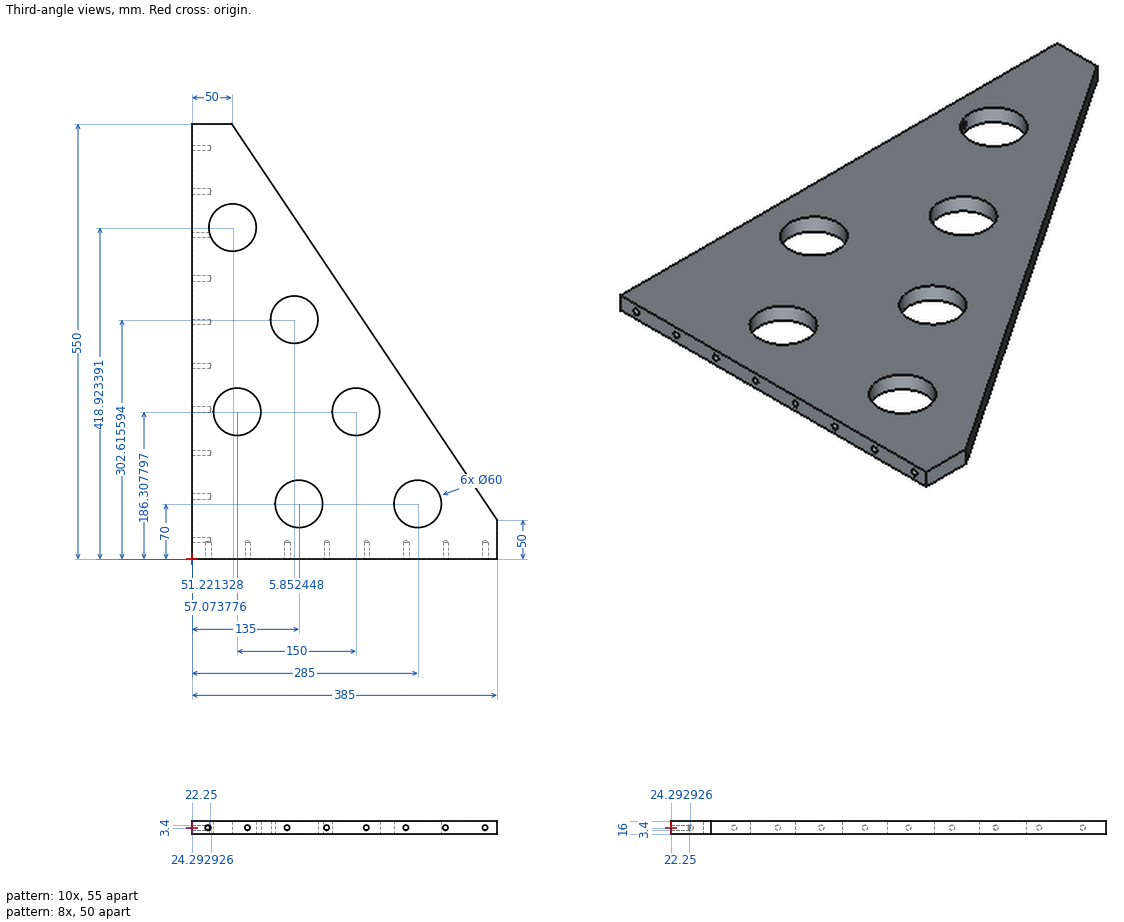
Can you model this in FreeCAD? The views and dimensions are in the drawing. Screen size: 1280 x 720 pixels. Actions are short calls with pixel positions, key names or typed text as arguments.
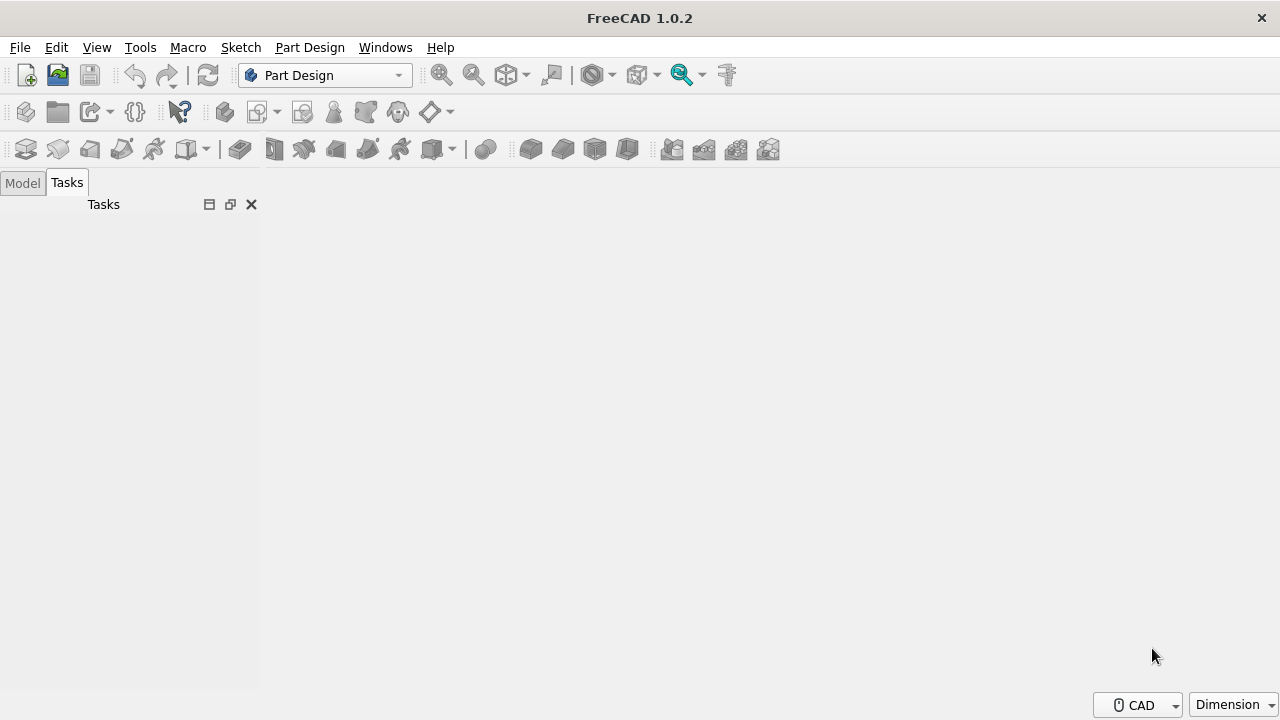
click(836, 112)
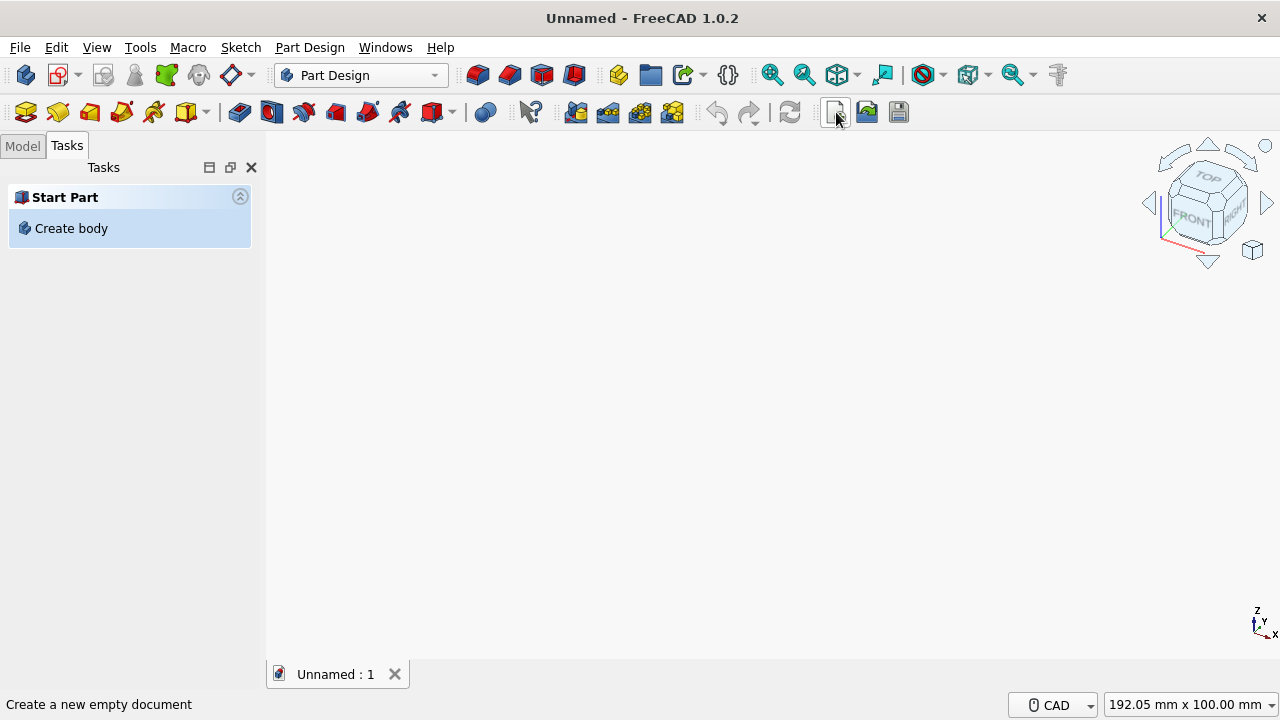
click(58, 76)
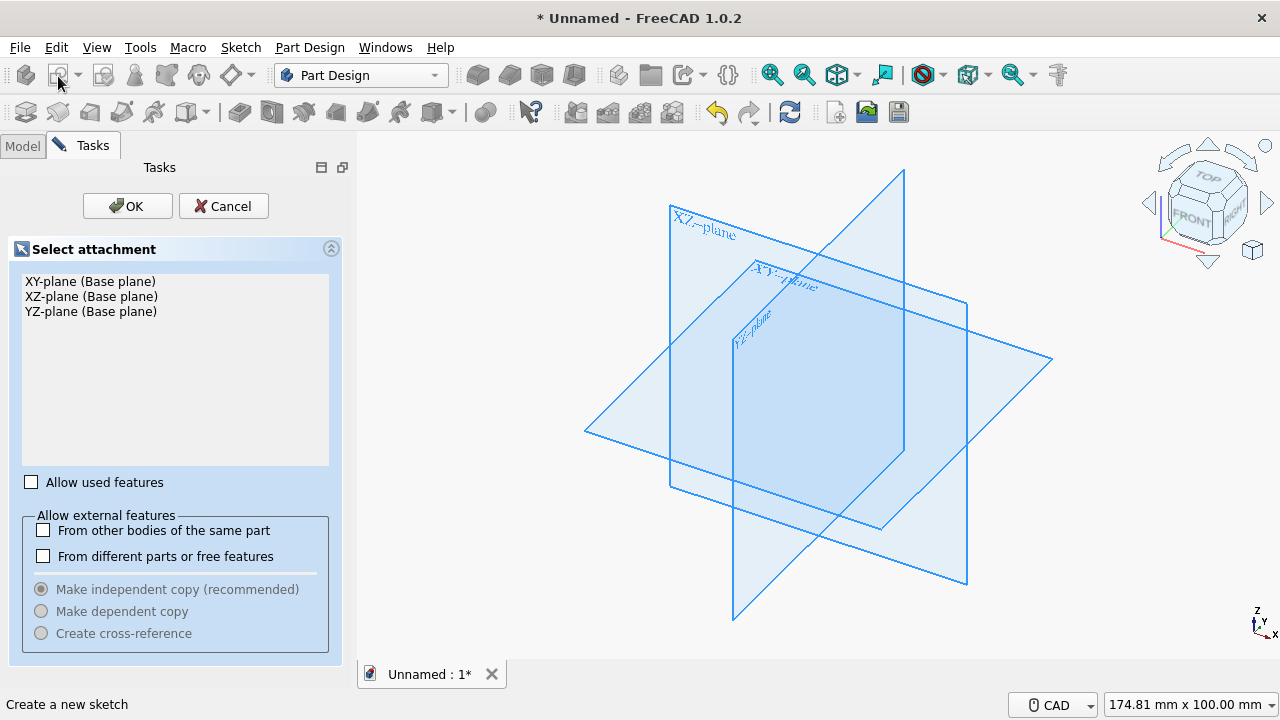
click(82, 282)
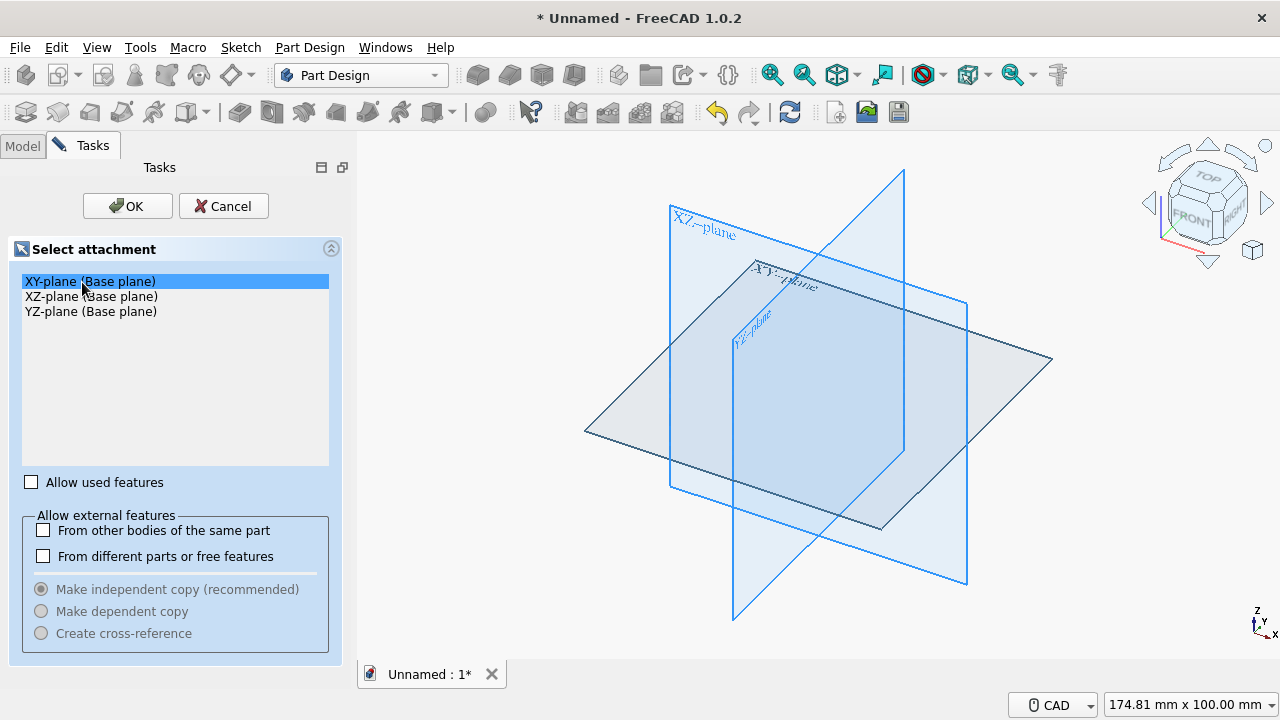
click(128, 206)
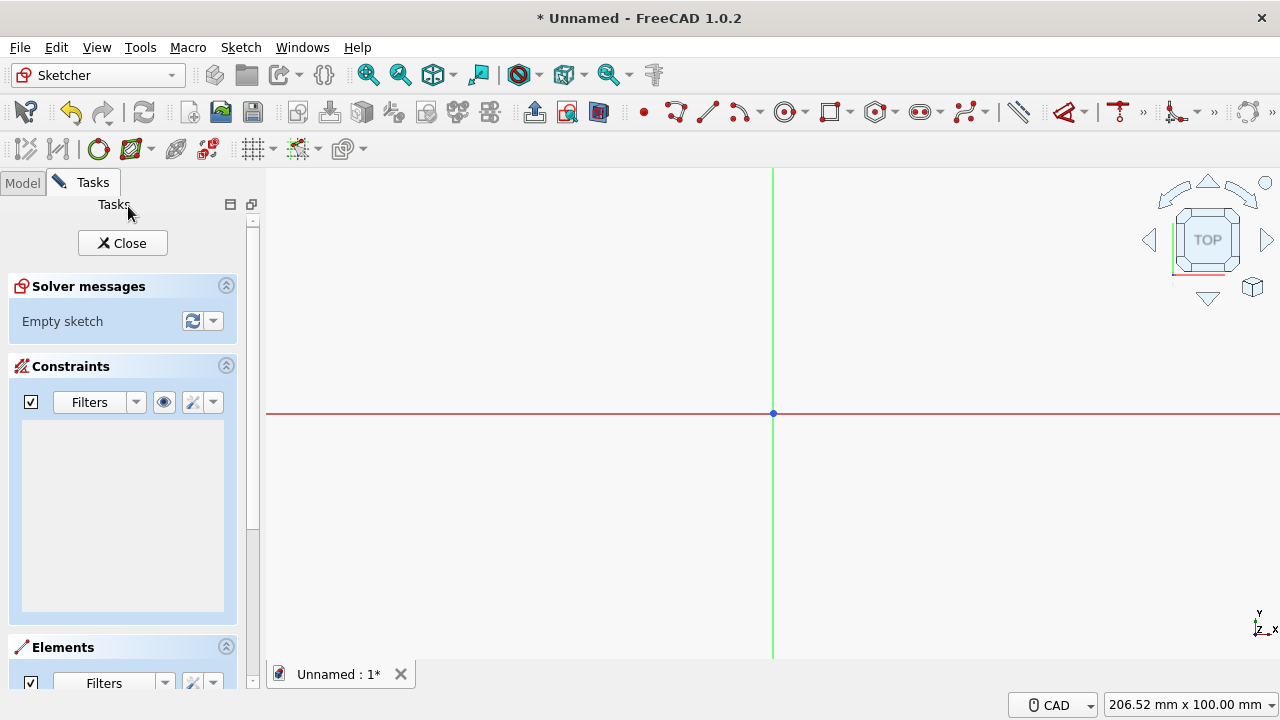
scroll(578, 582, down, 11)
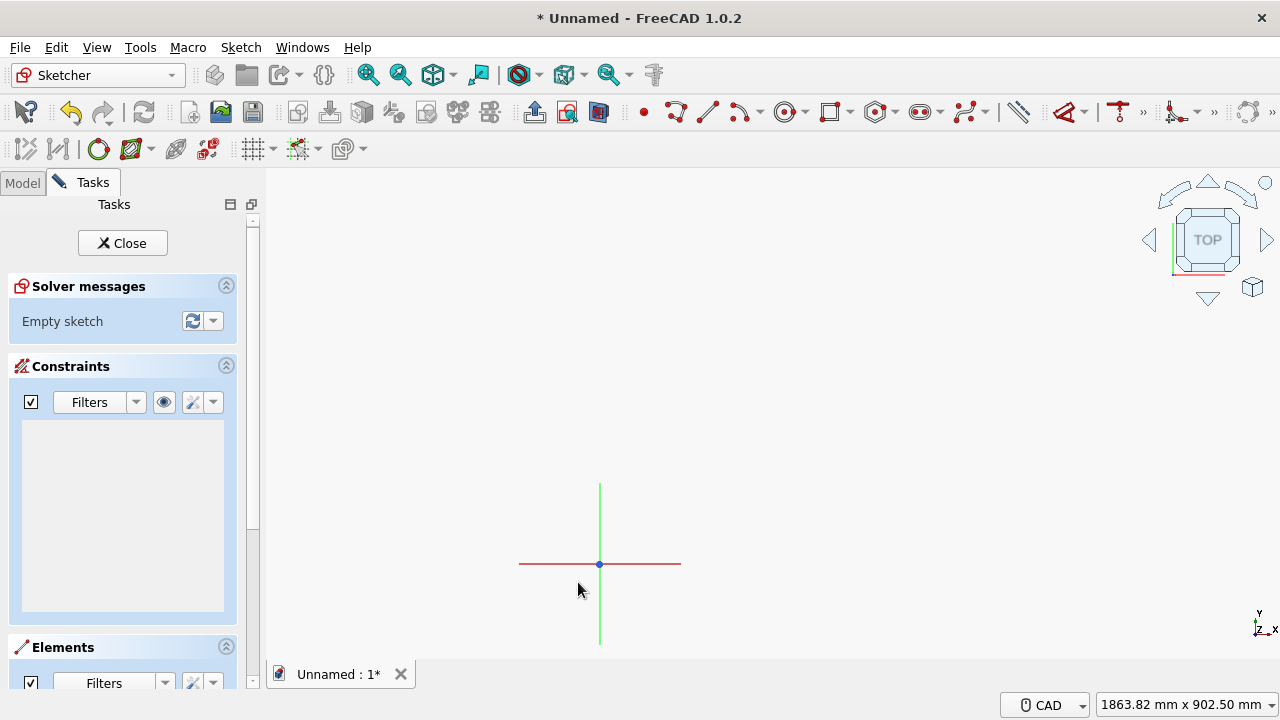
click(676, 112)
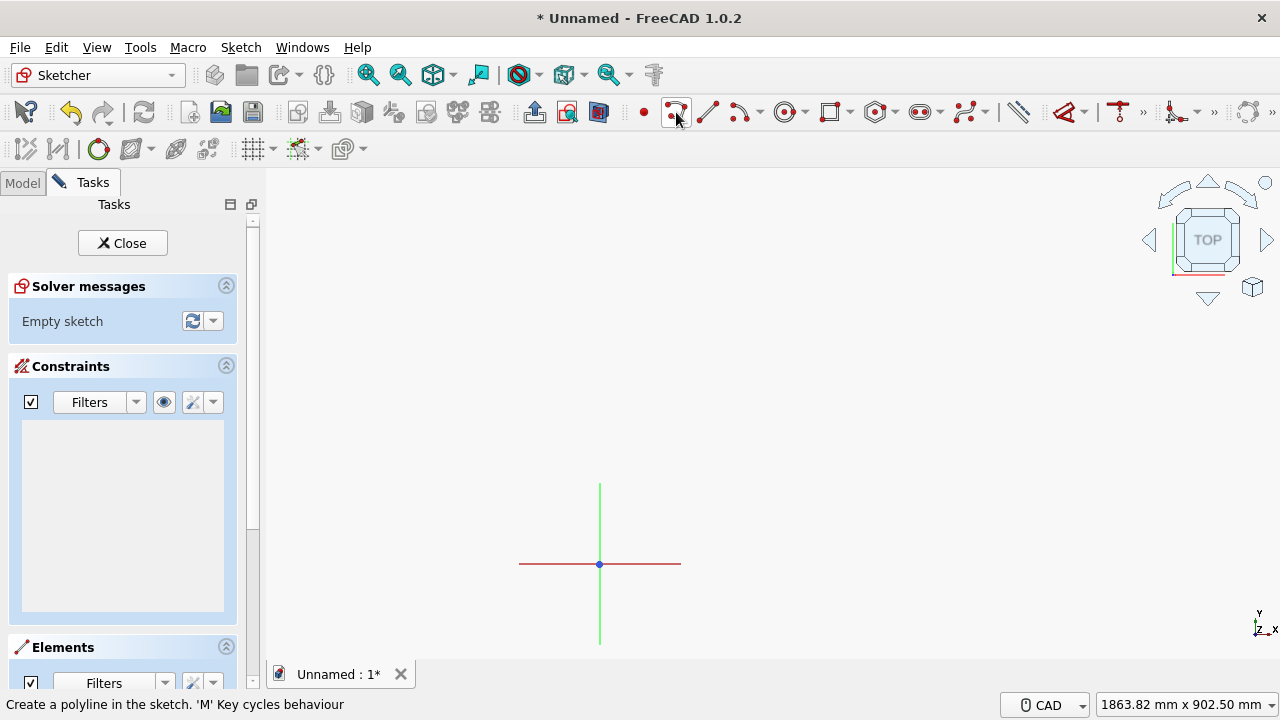
click(600, 564)
click(809, 555)
click(809, 537)
click(627, 265)
click(609, 265)
click(600, 564)
key(Escape)
key(Escape)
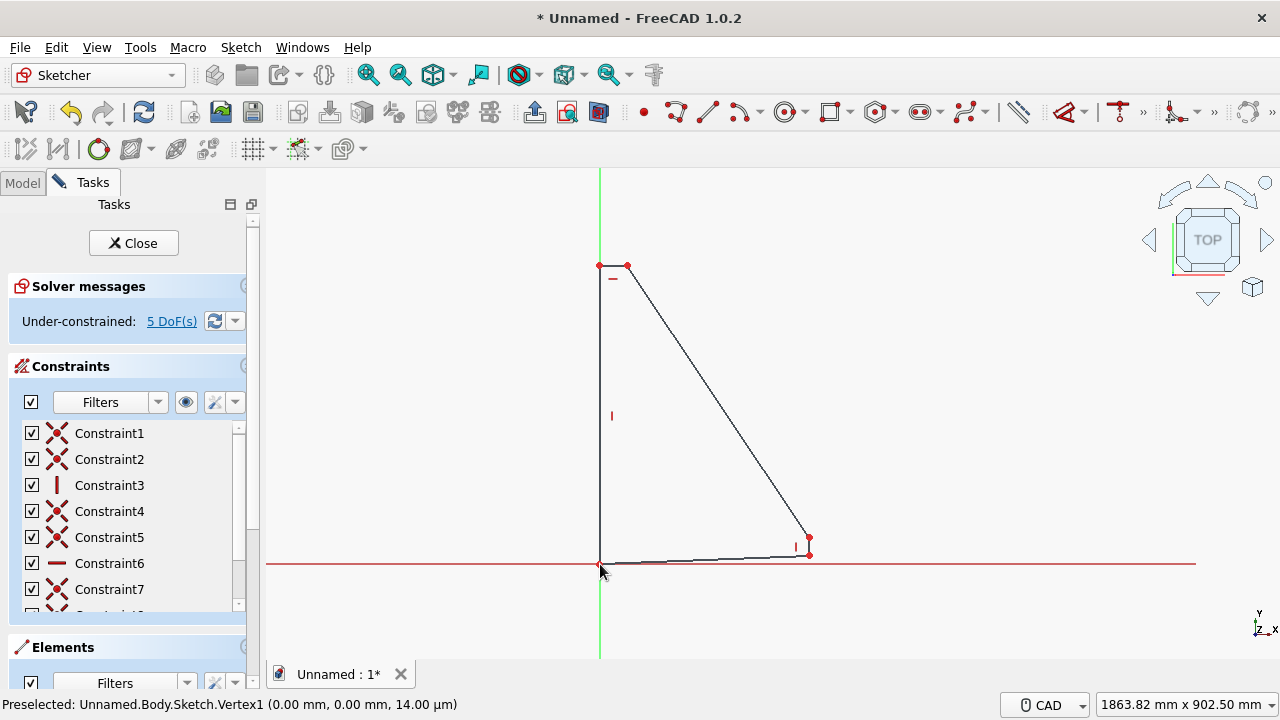
click(663, 562)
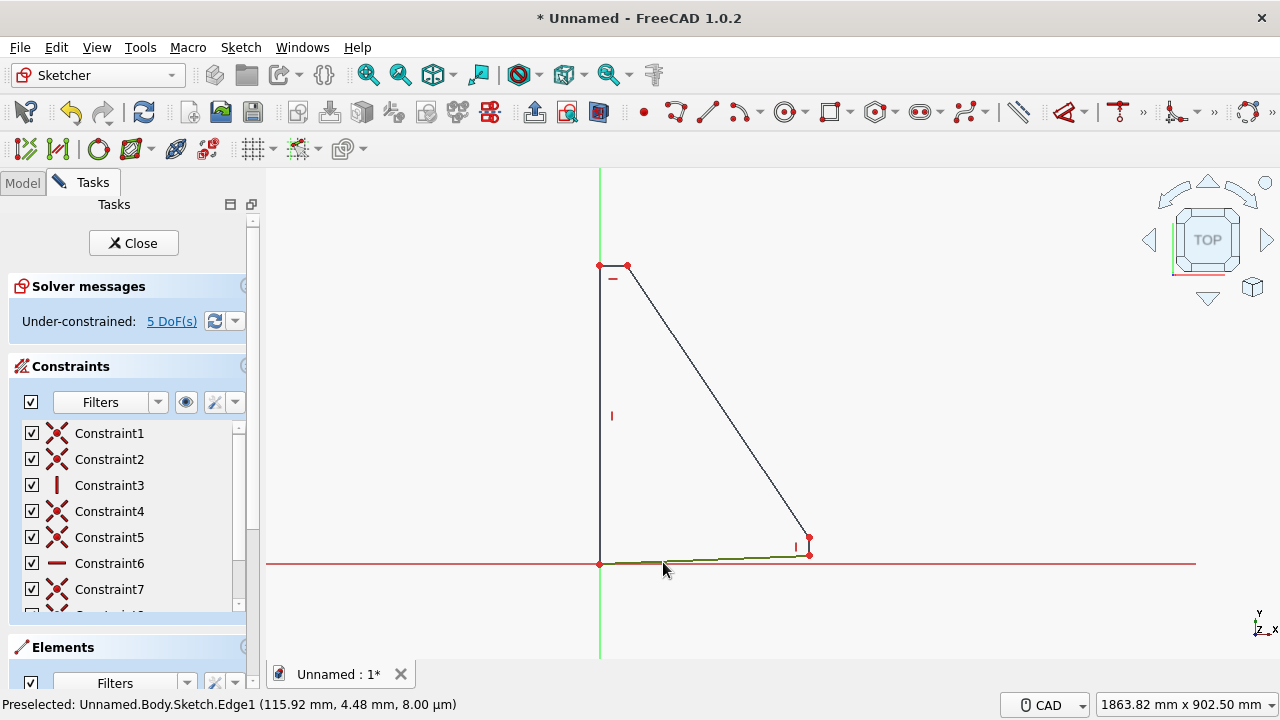
key(h)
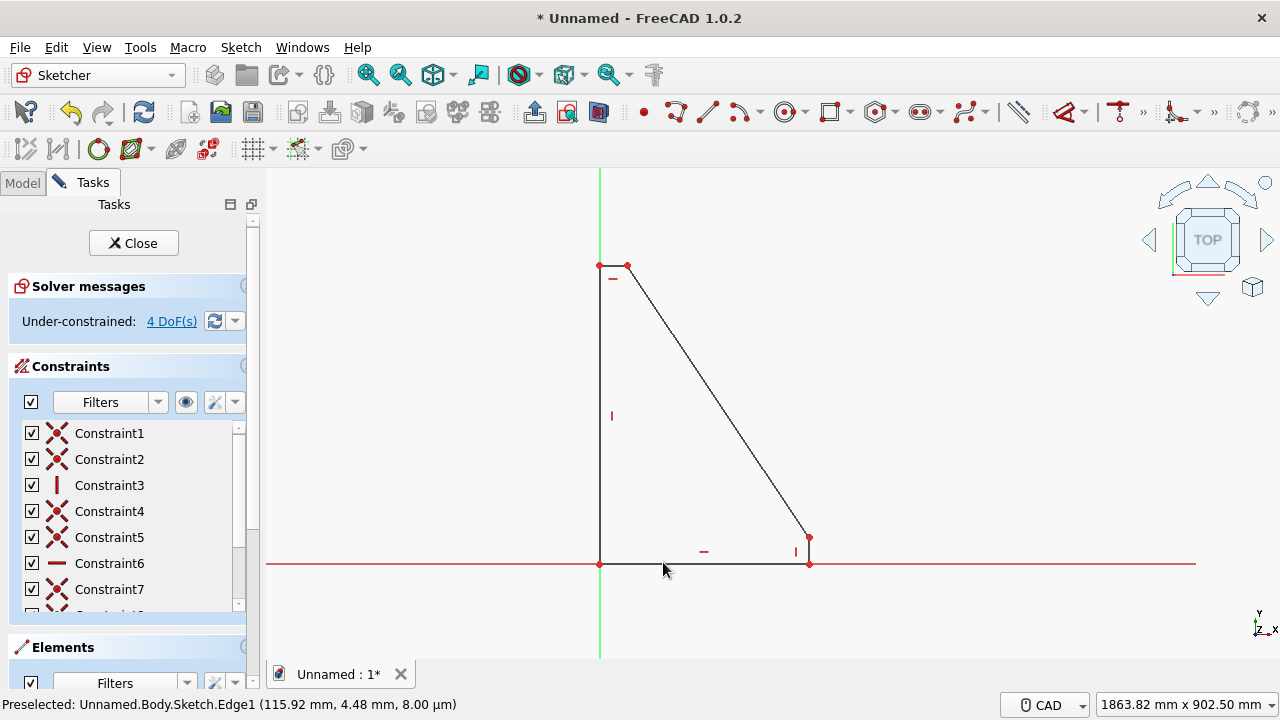
scroll(809, 554, up, 2)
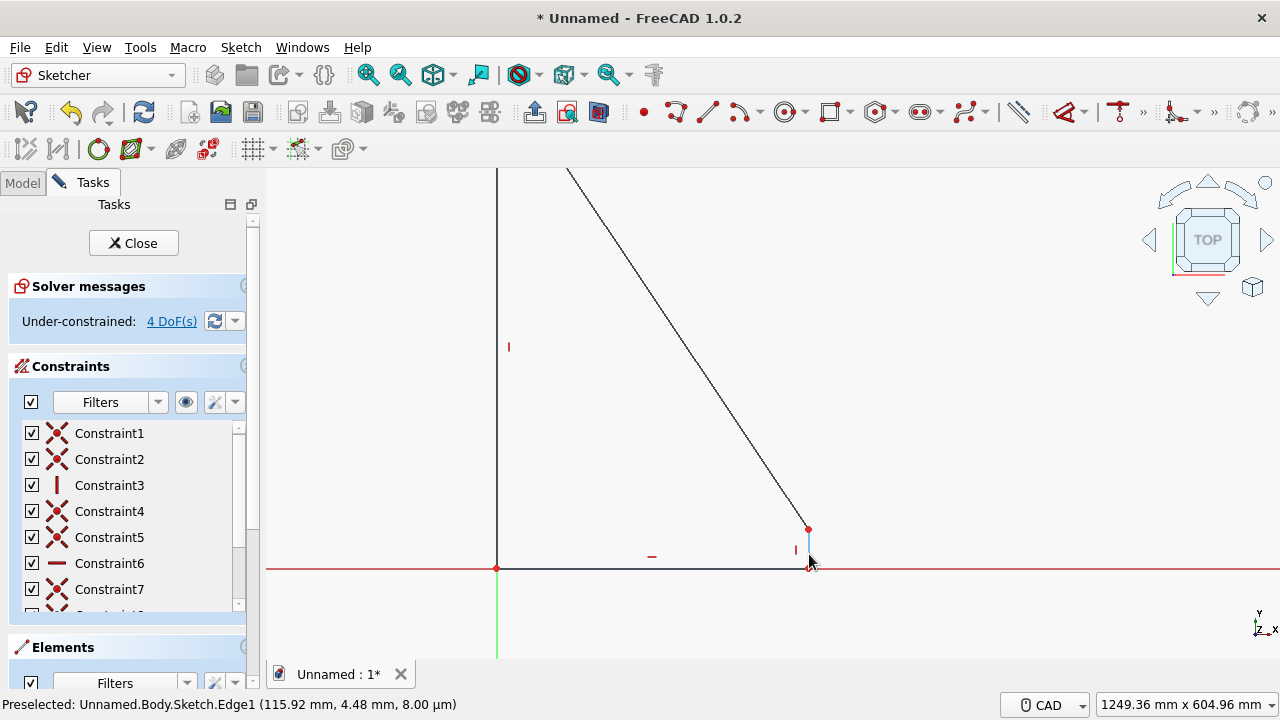
click(809, 553)